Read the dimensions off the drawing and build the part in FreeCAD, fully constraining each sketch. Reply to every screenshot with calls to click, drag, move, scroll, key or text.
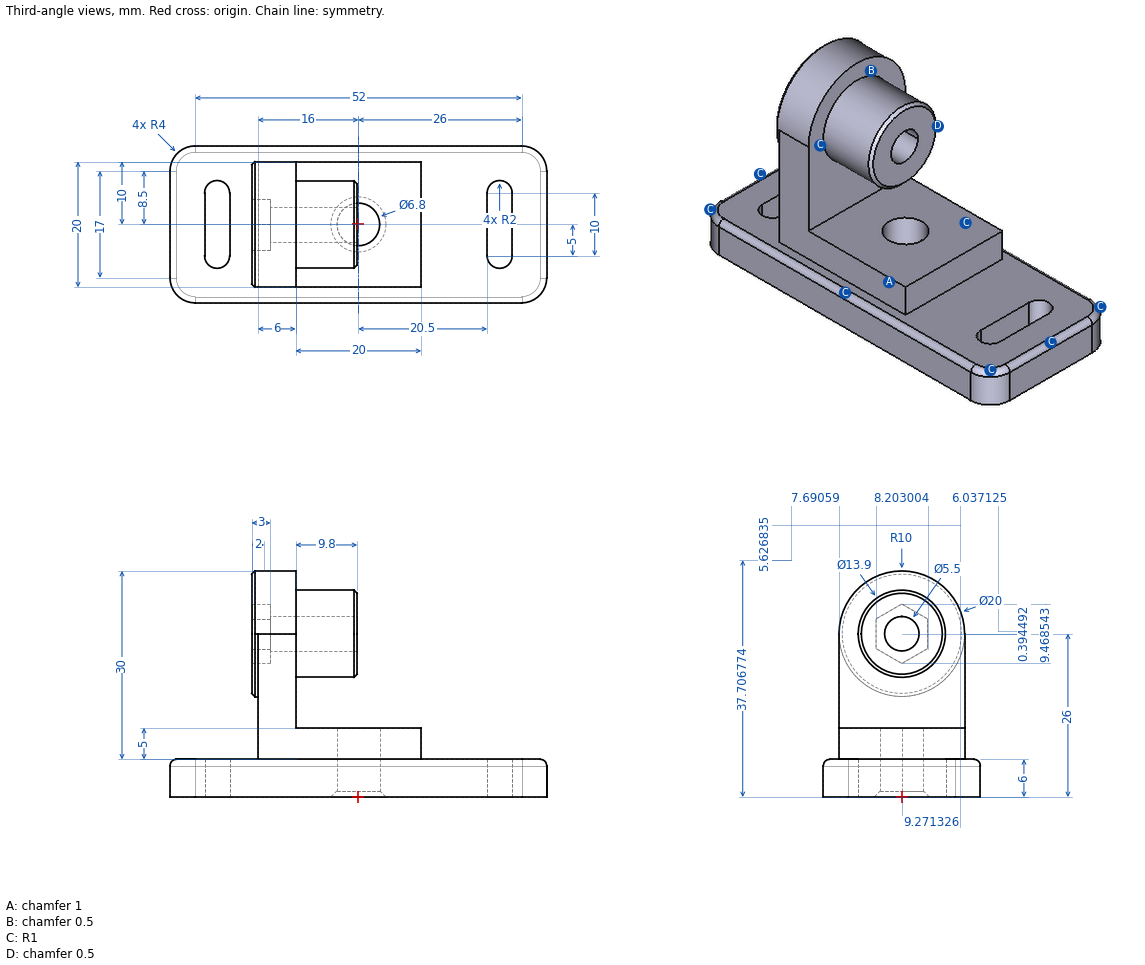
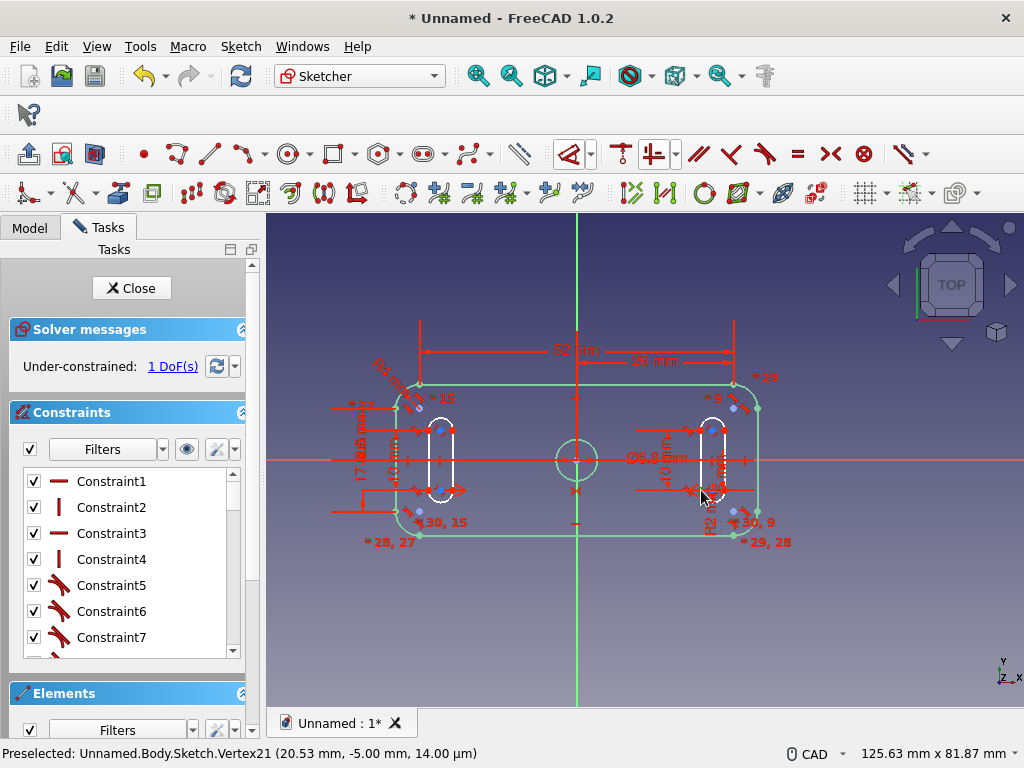
key(l)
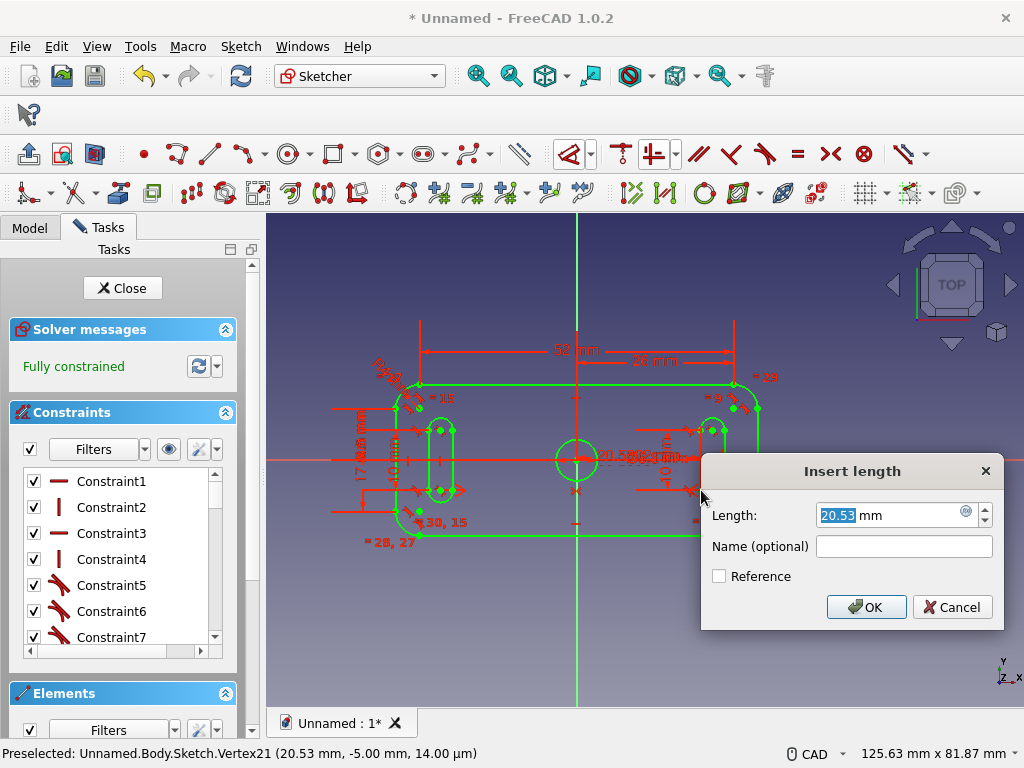
text(20.5)
key(Return)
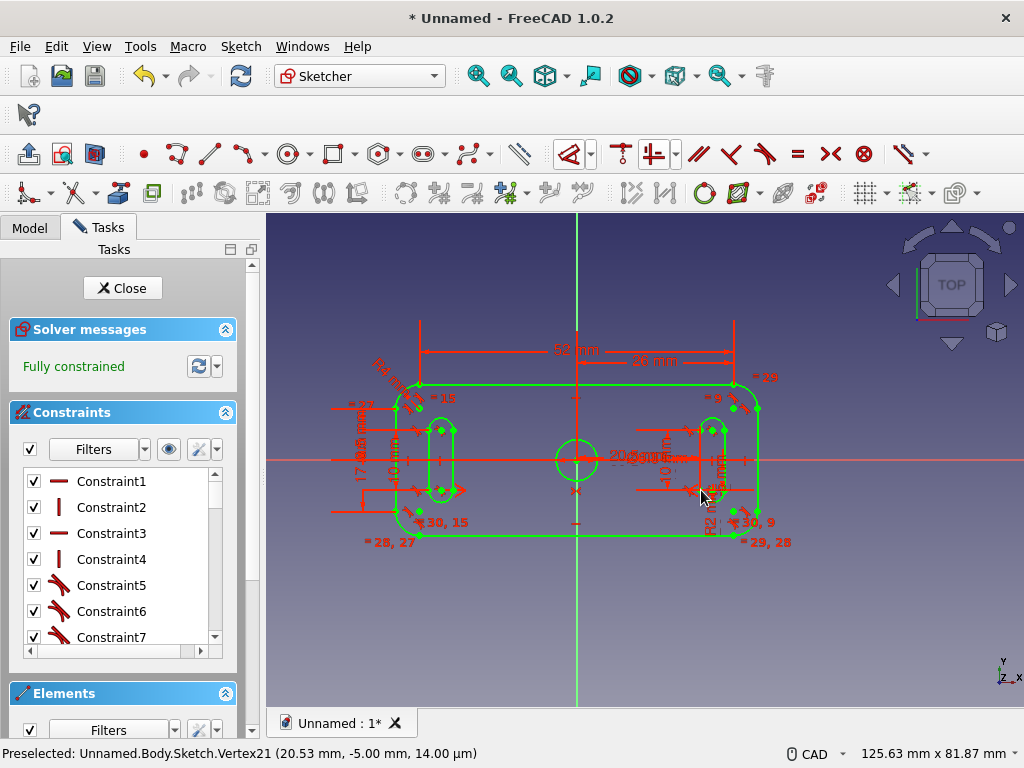
click(123, 288)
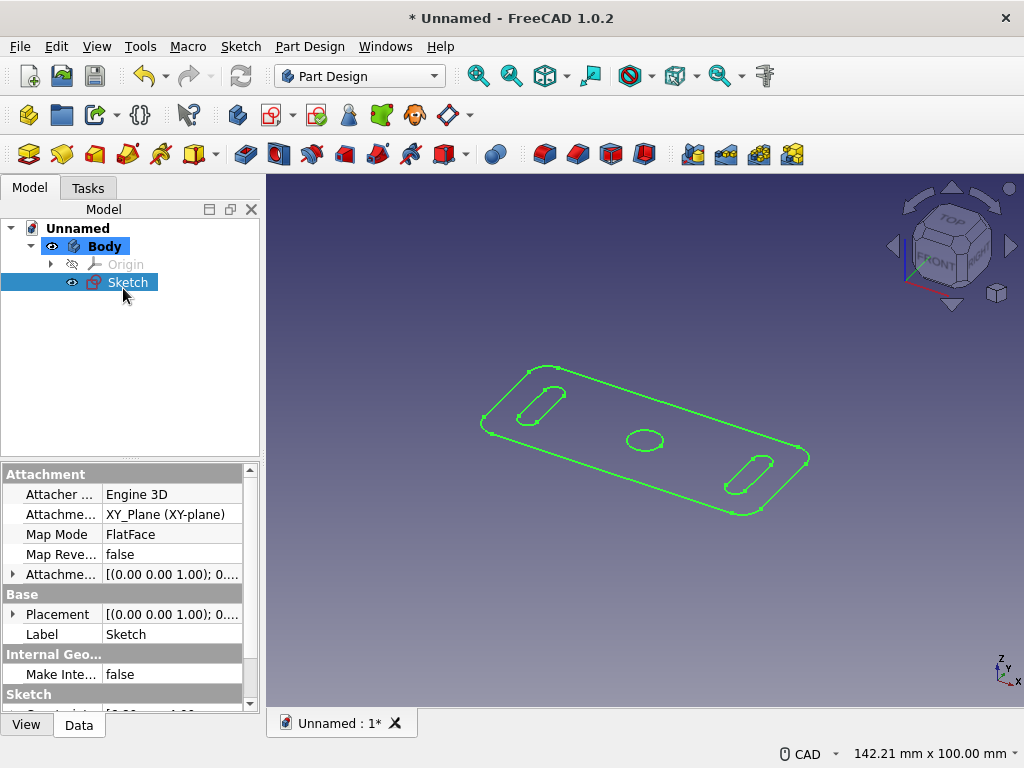
click(29, 154)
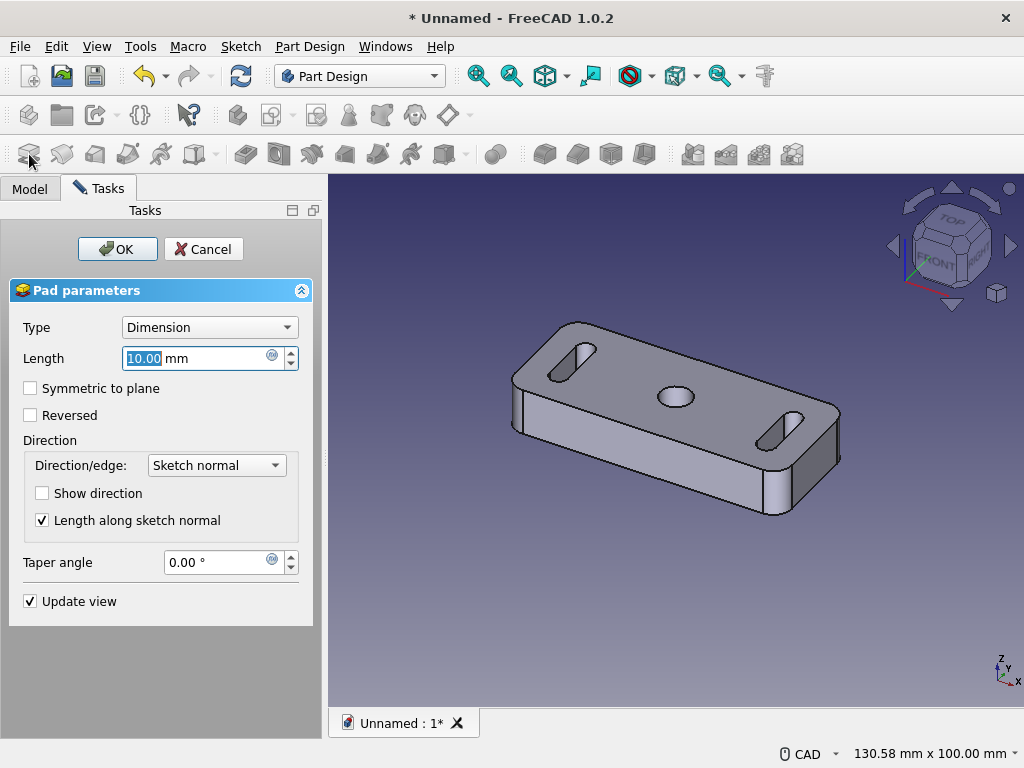
text(6)
key(Tab)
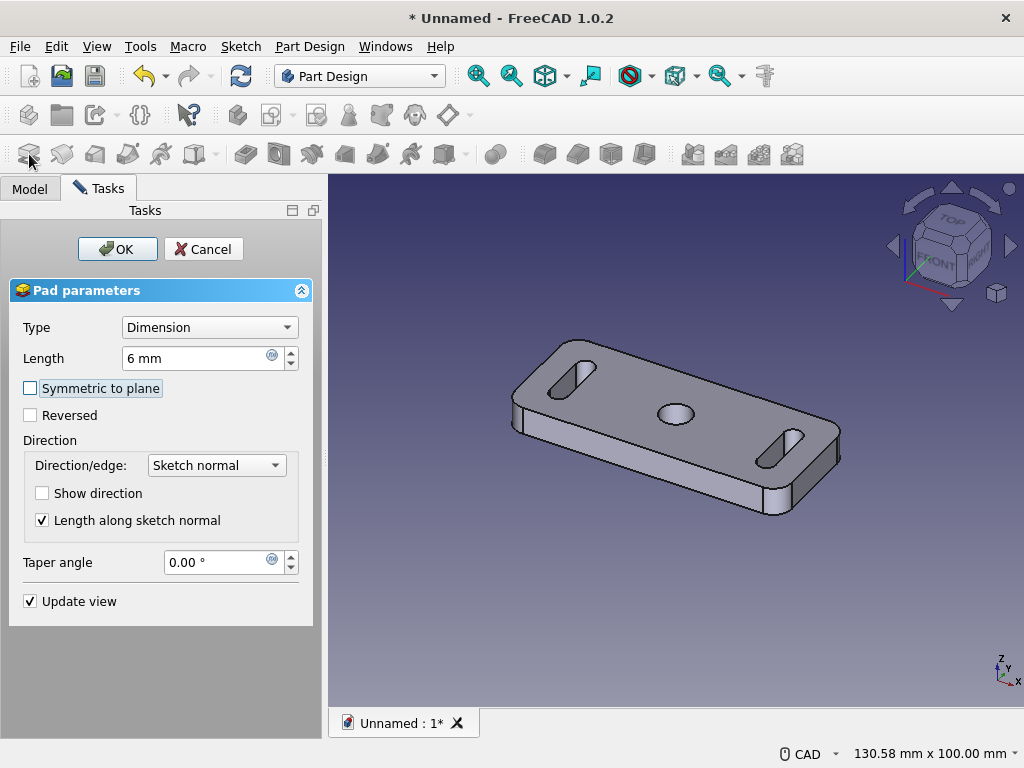
click(118, 249)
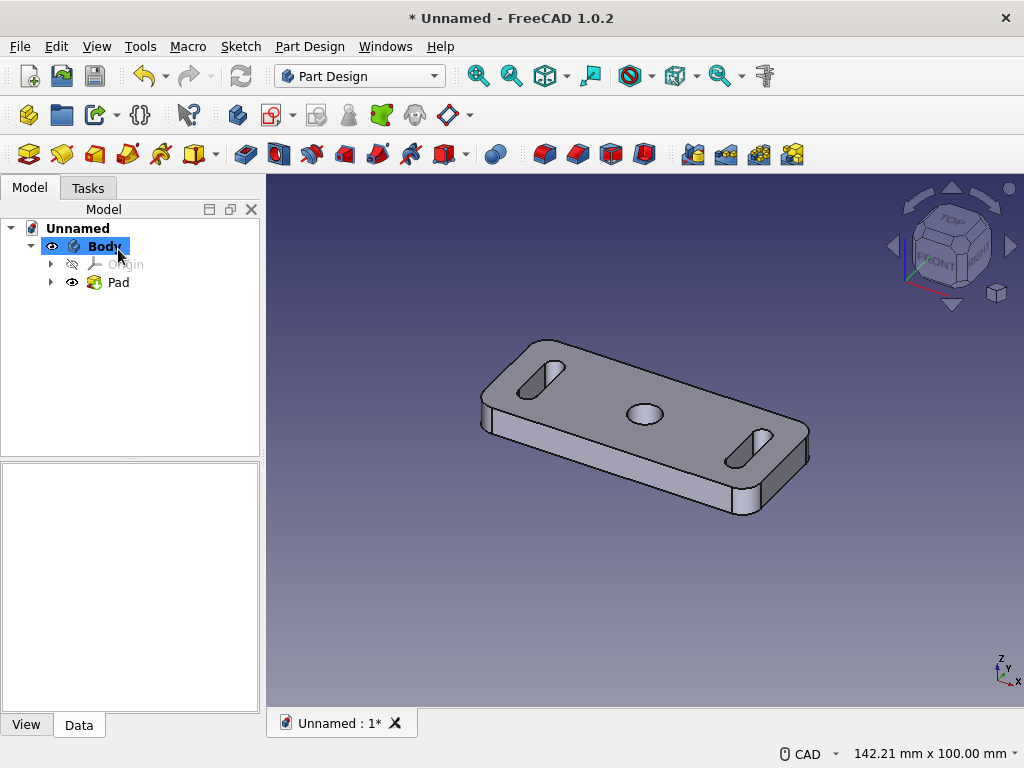
key(0)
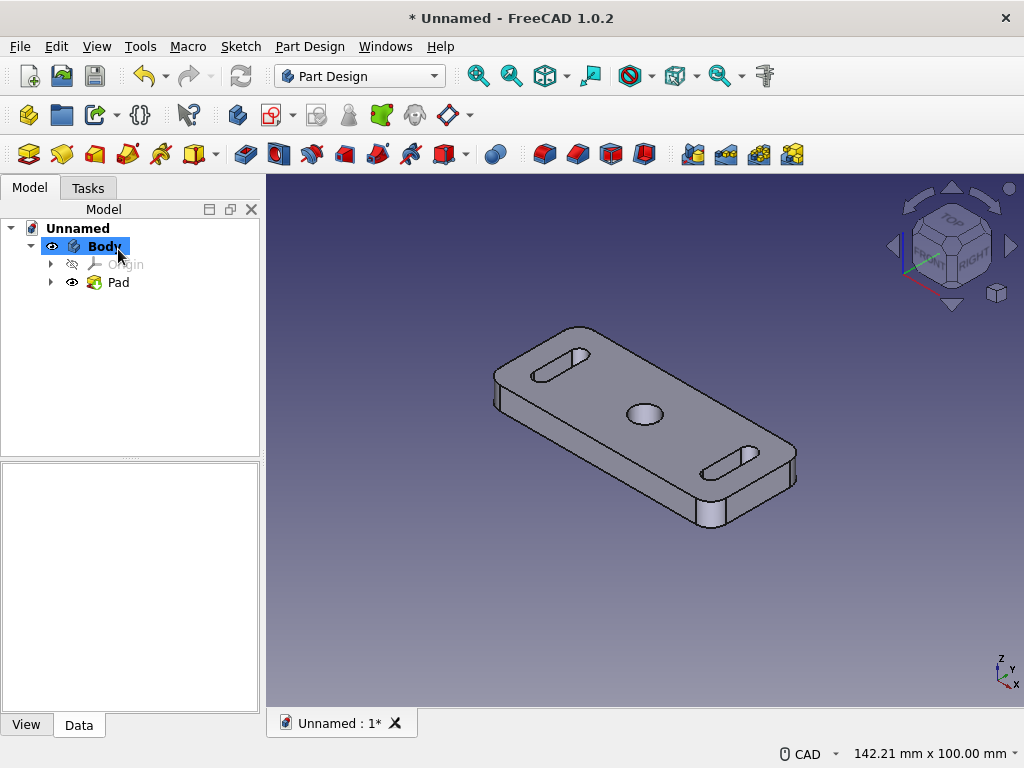
click(479, 76)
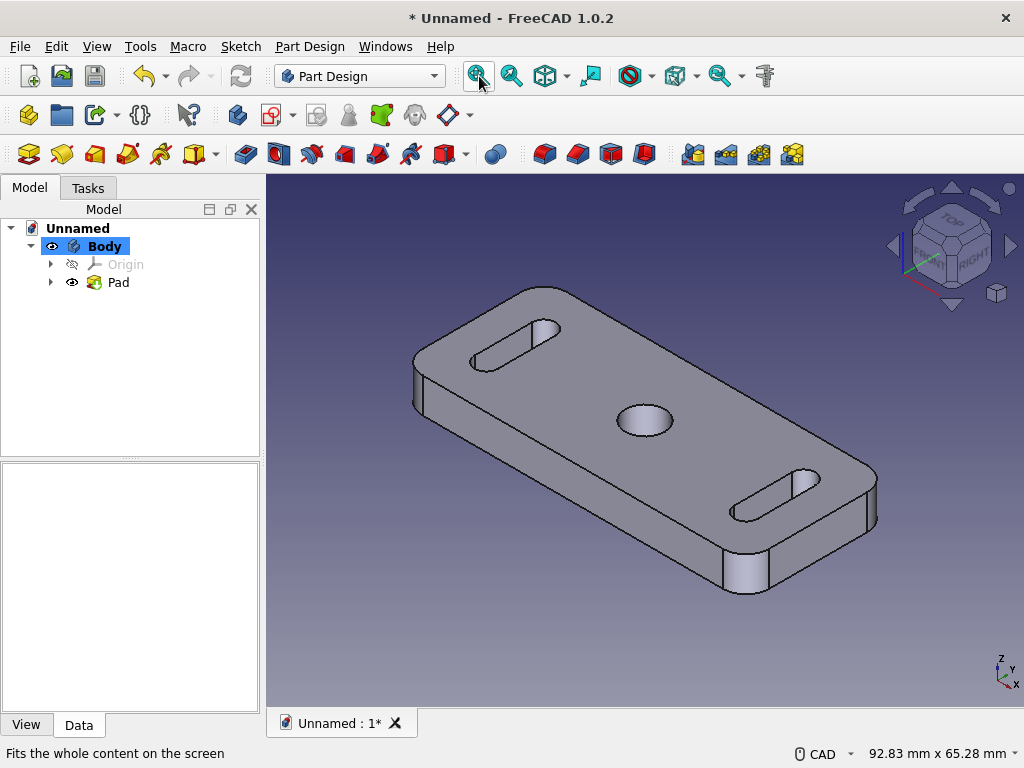
key(2)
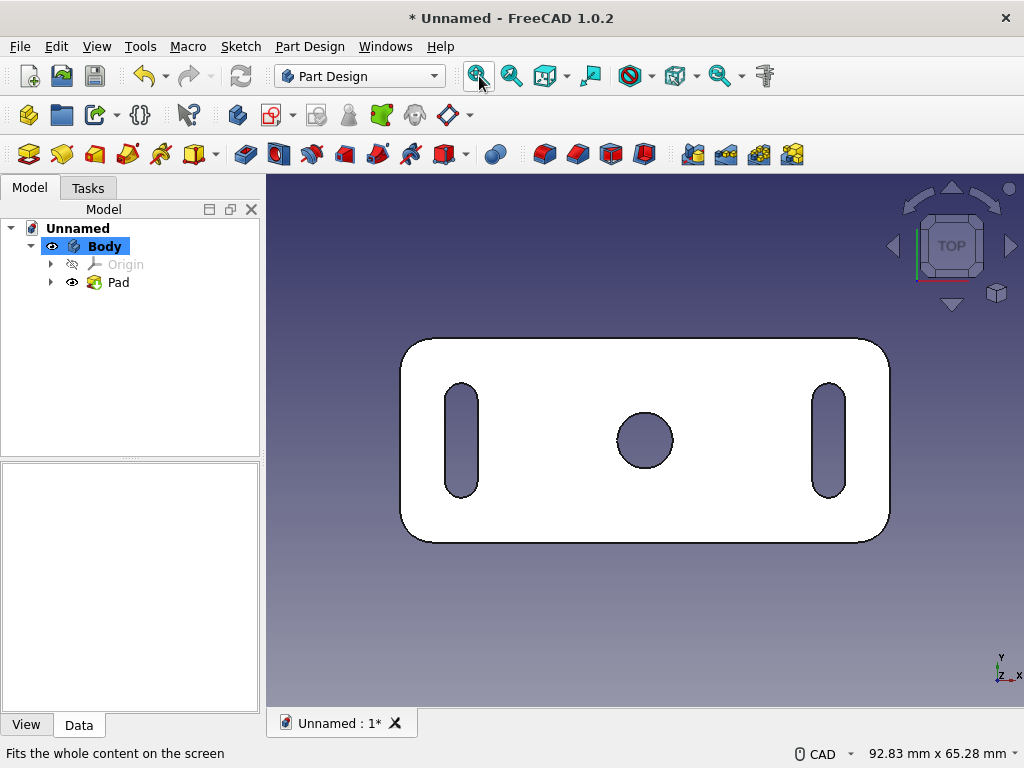
key(1)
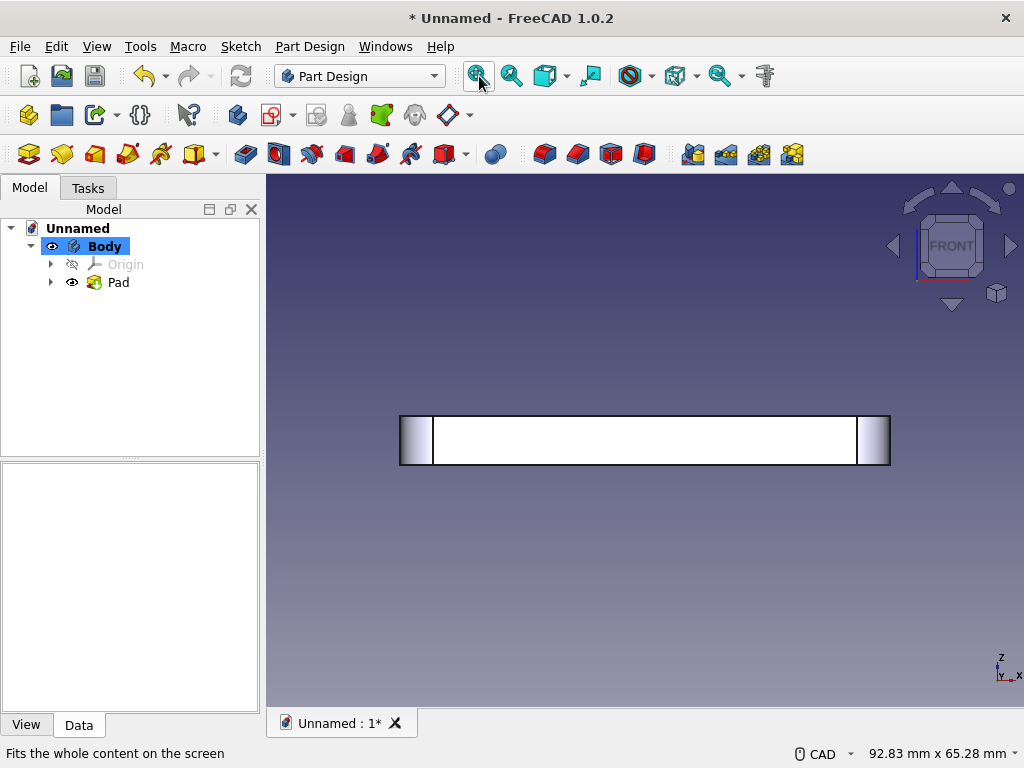
key(3)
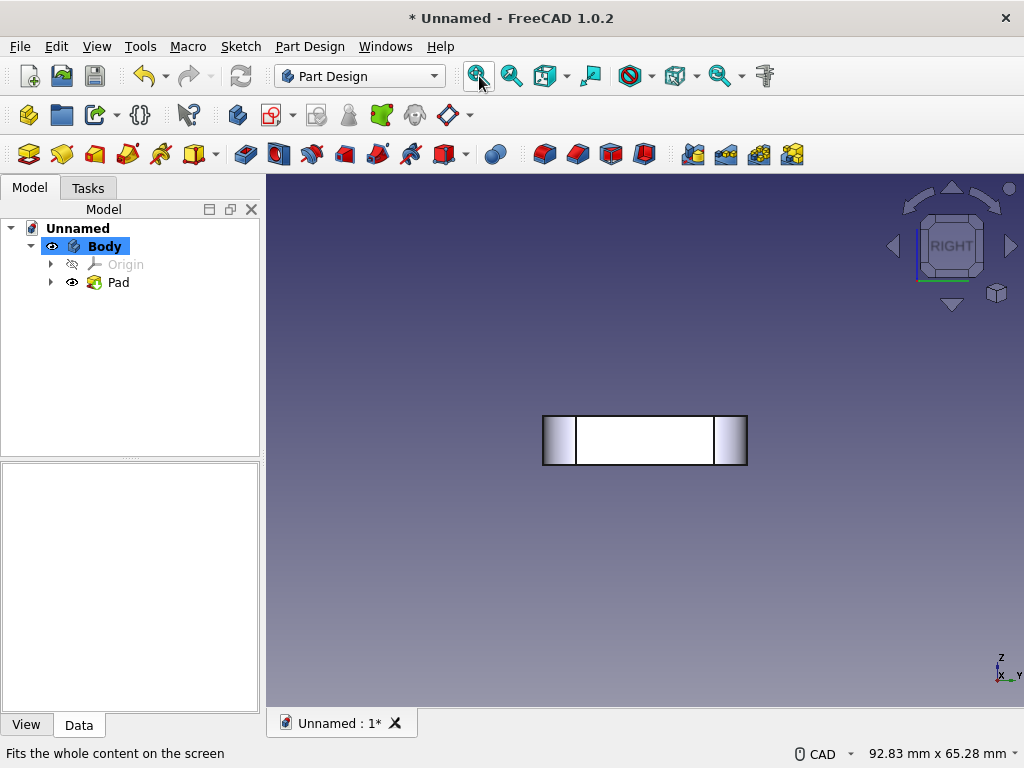
click(479, 76)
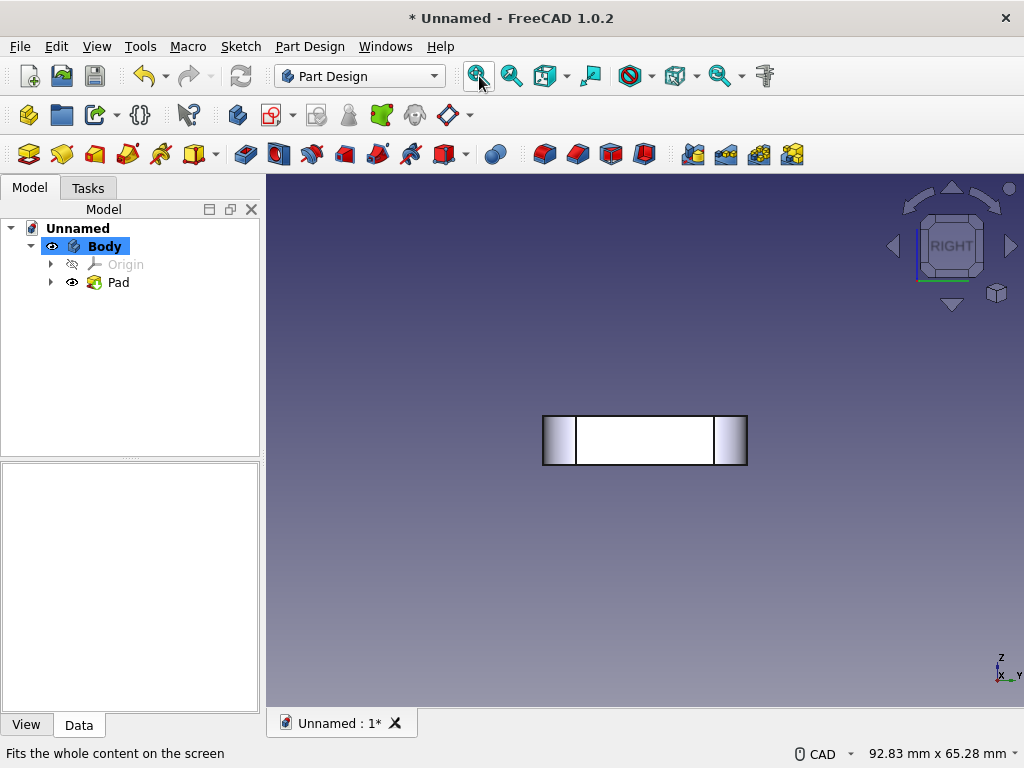
key(5)